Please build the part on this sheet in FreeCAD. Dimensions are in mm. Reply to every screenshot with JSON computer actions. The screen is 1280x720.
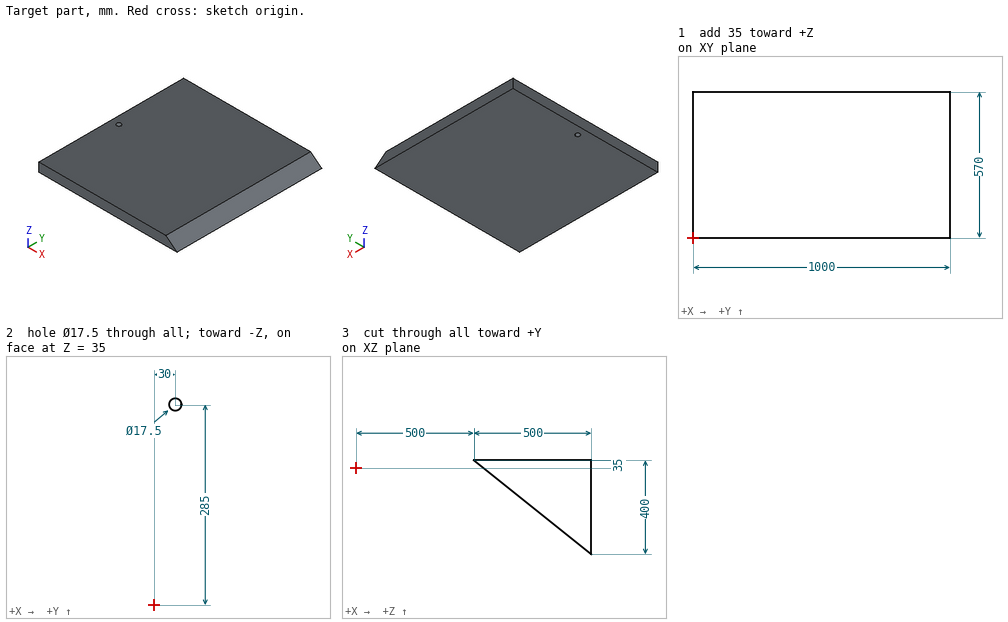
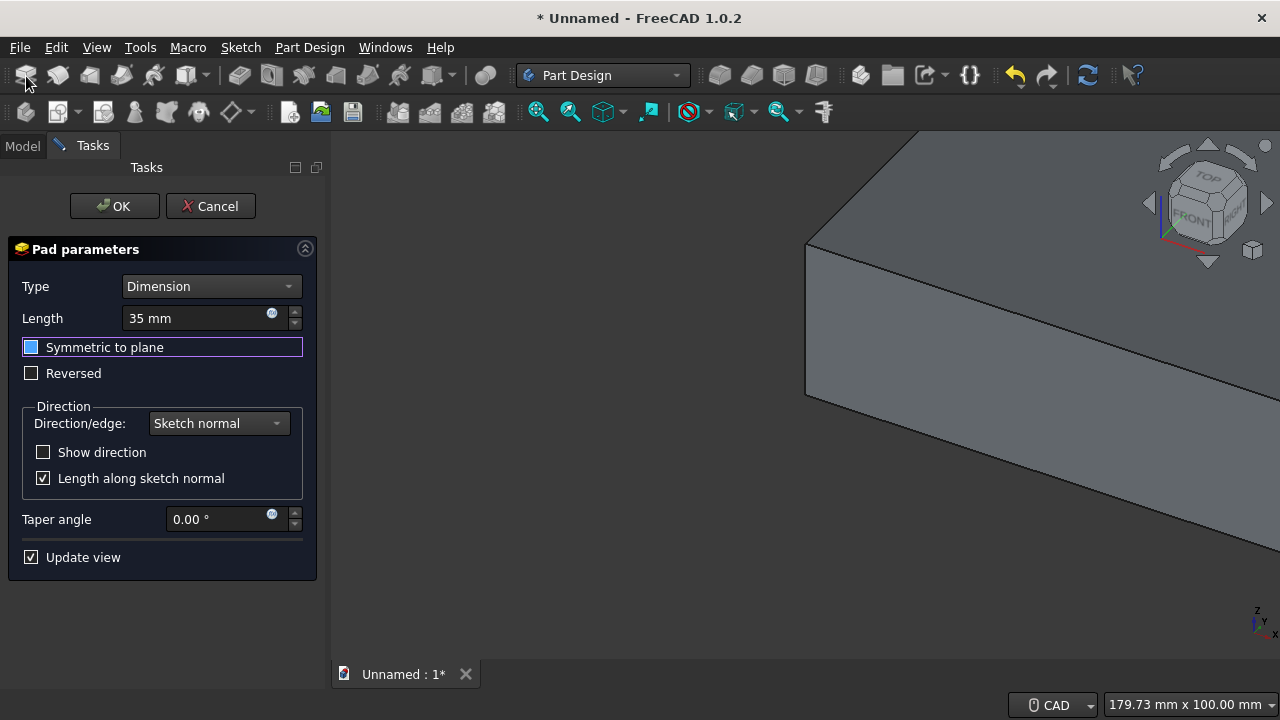
{"action": "left_click", "coordinate": [115, 206]}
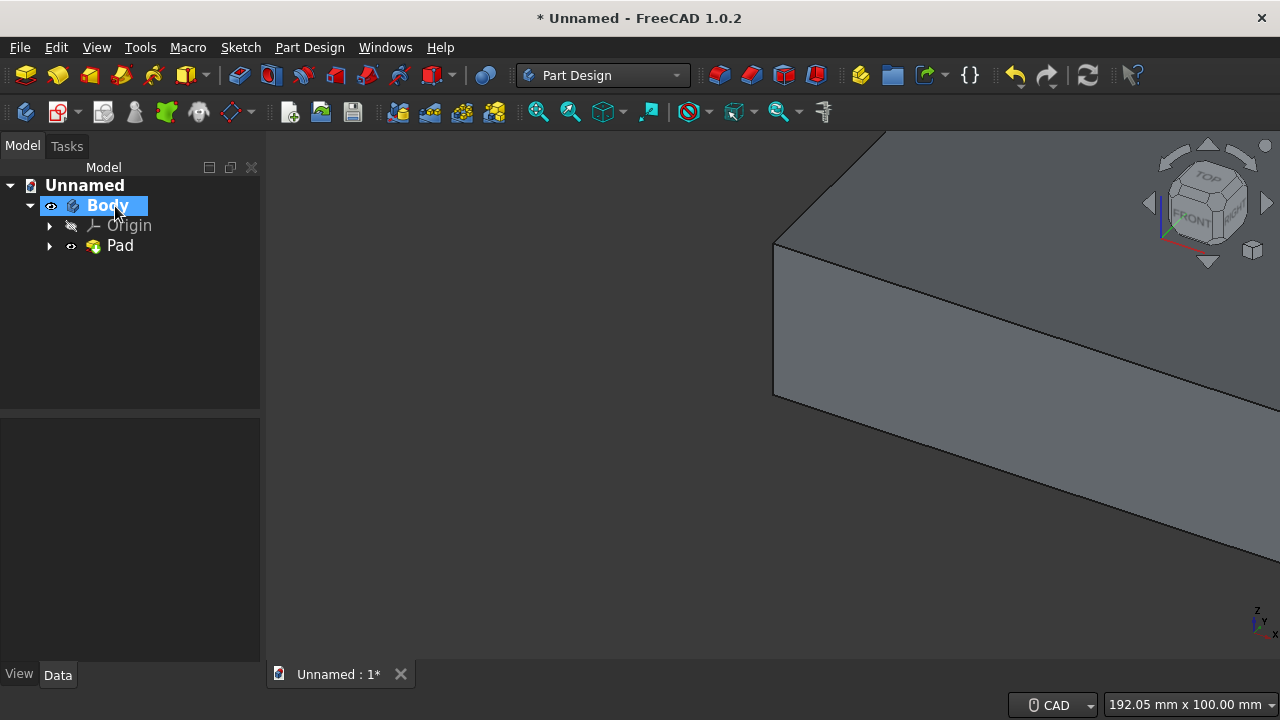
{"action": "key", "text": "v f"}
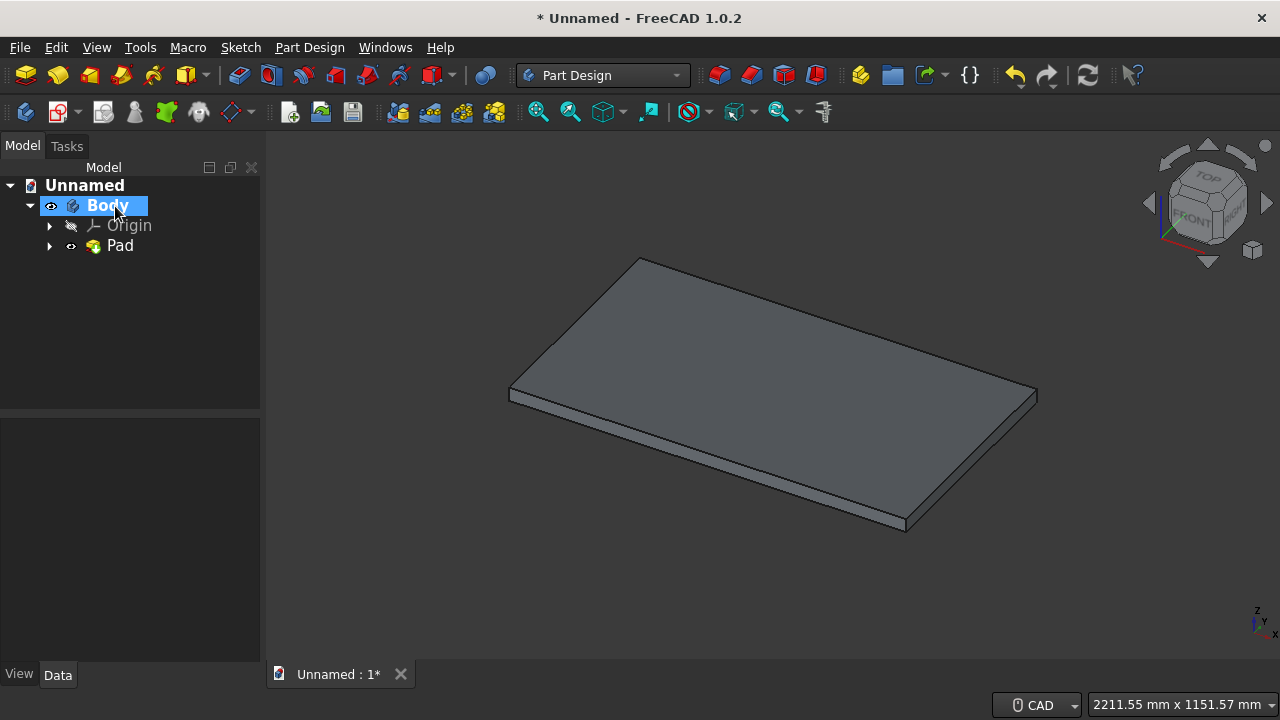
{"action": "left_click", "coordinate": [830, 406]}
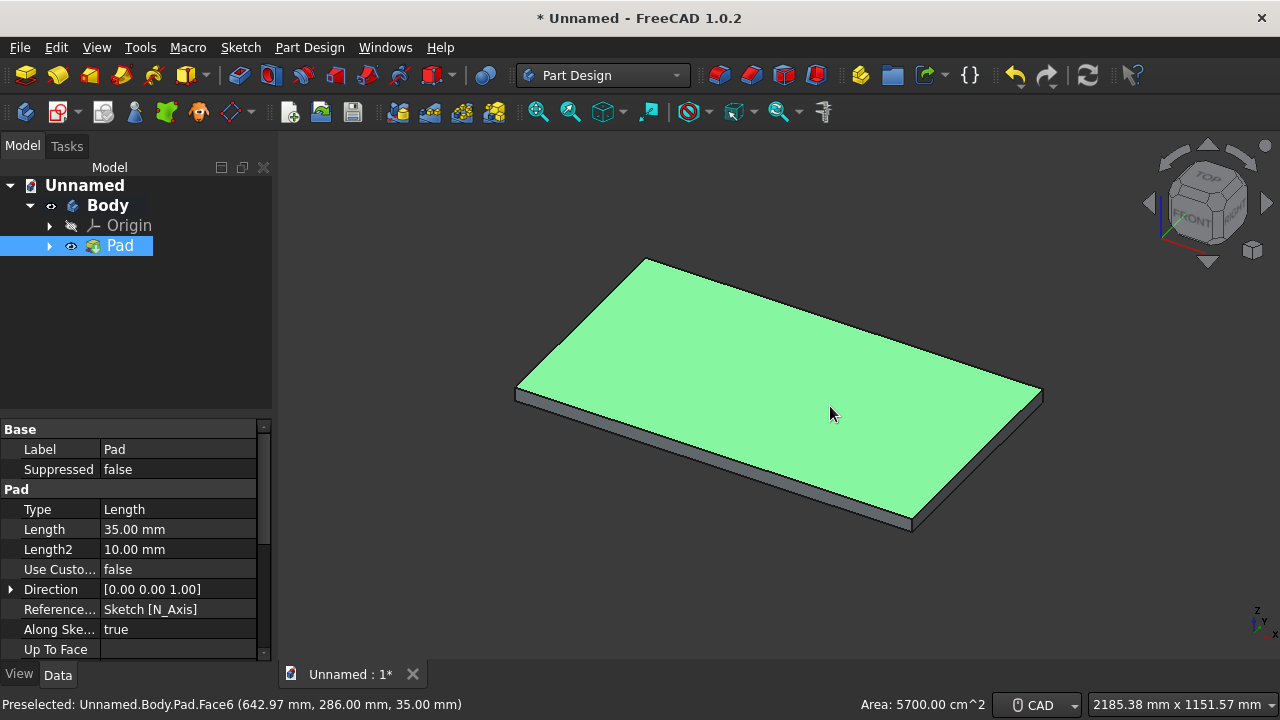
{"action": "left_click", "coordinate": [58, 112]}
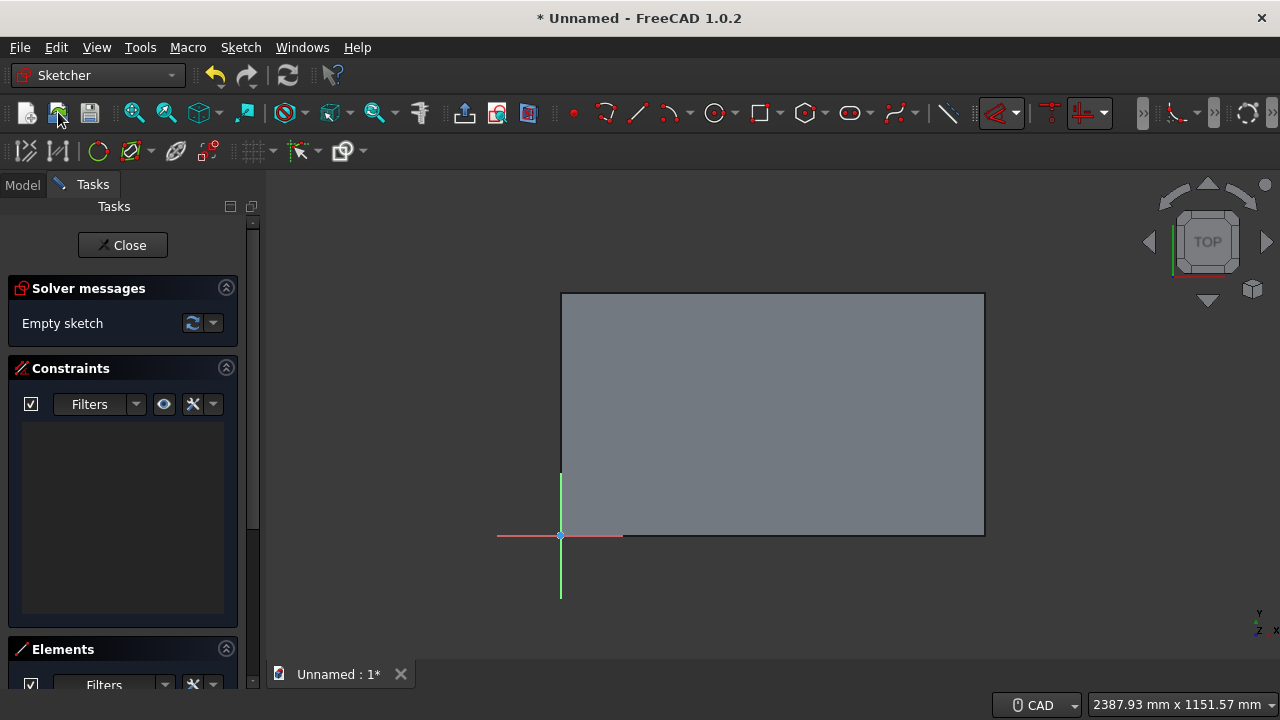
{"action": "scroll", "coordinate": [567, 414], "scroll_direction": "up", "scroll_amount": 15}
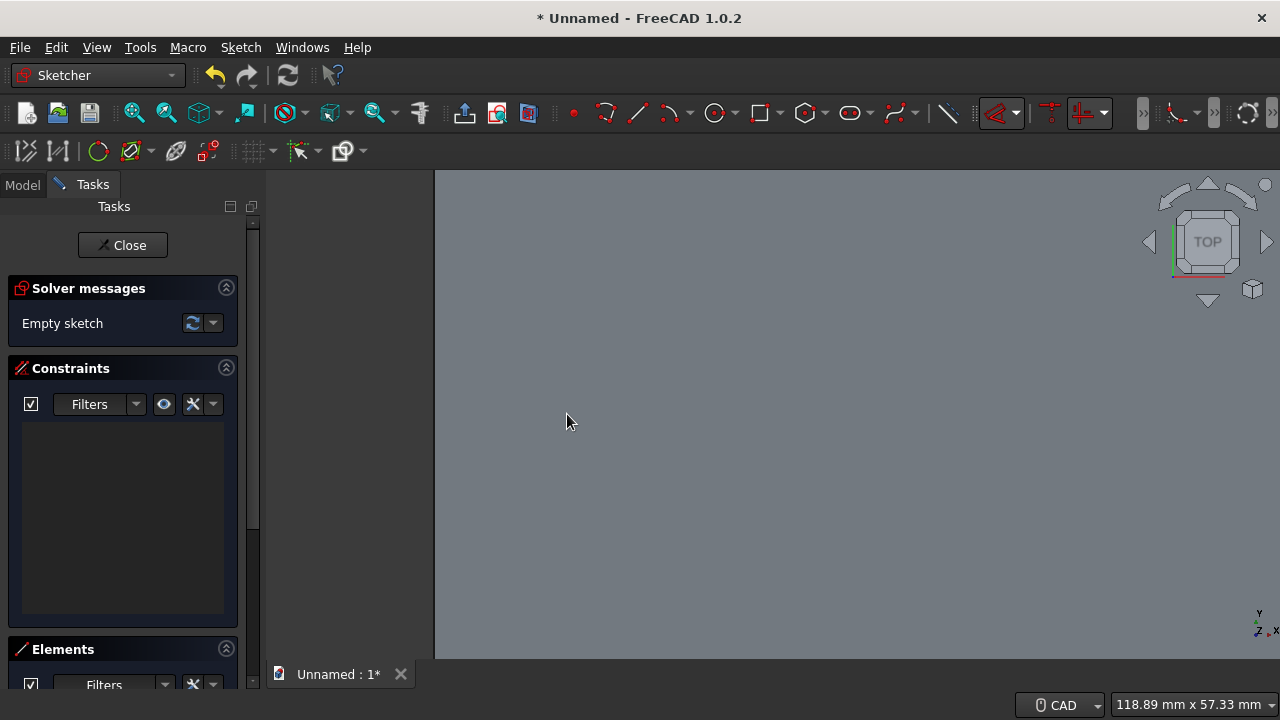
{"action": "scroll", "coordinate": [679, 414], "scroll_direction": "up", "scroll_amount": 4}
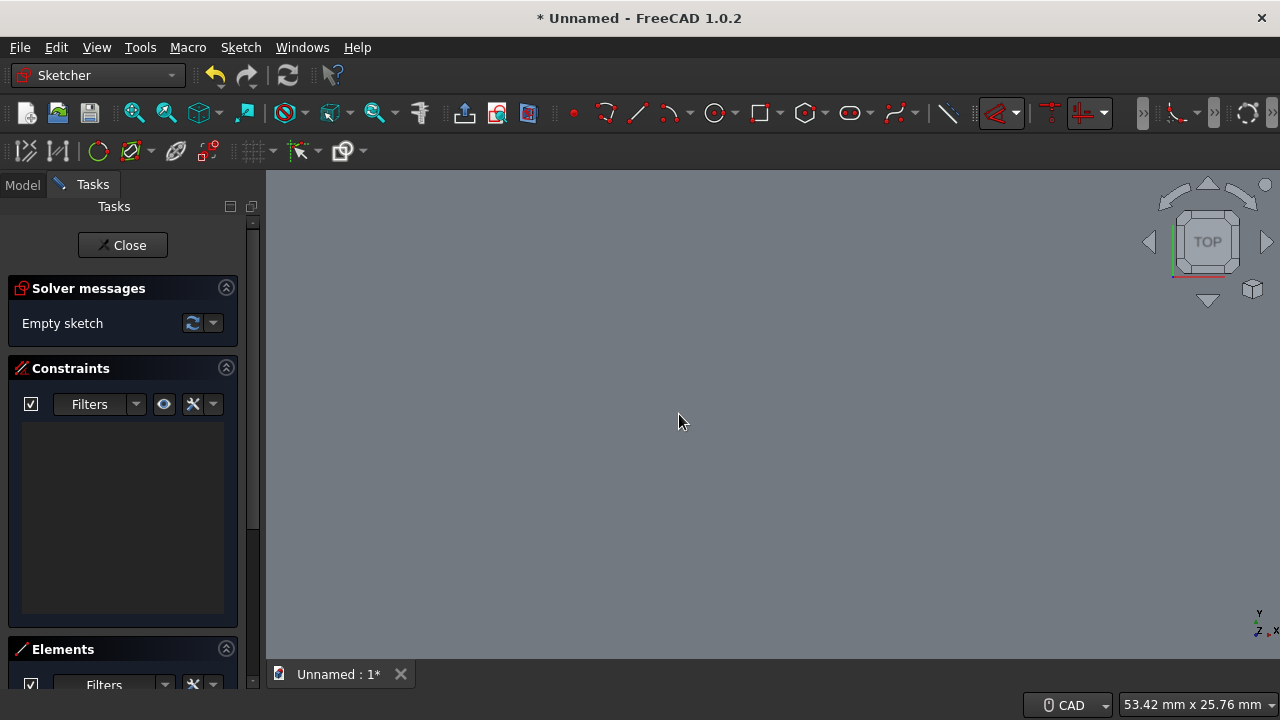
{"action": "left_click", "coordinate": [716, 114]}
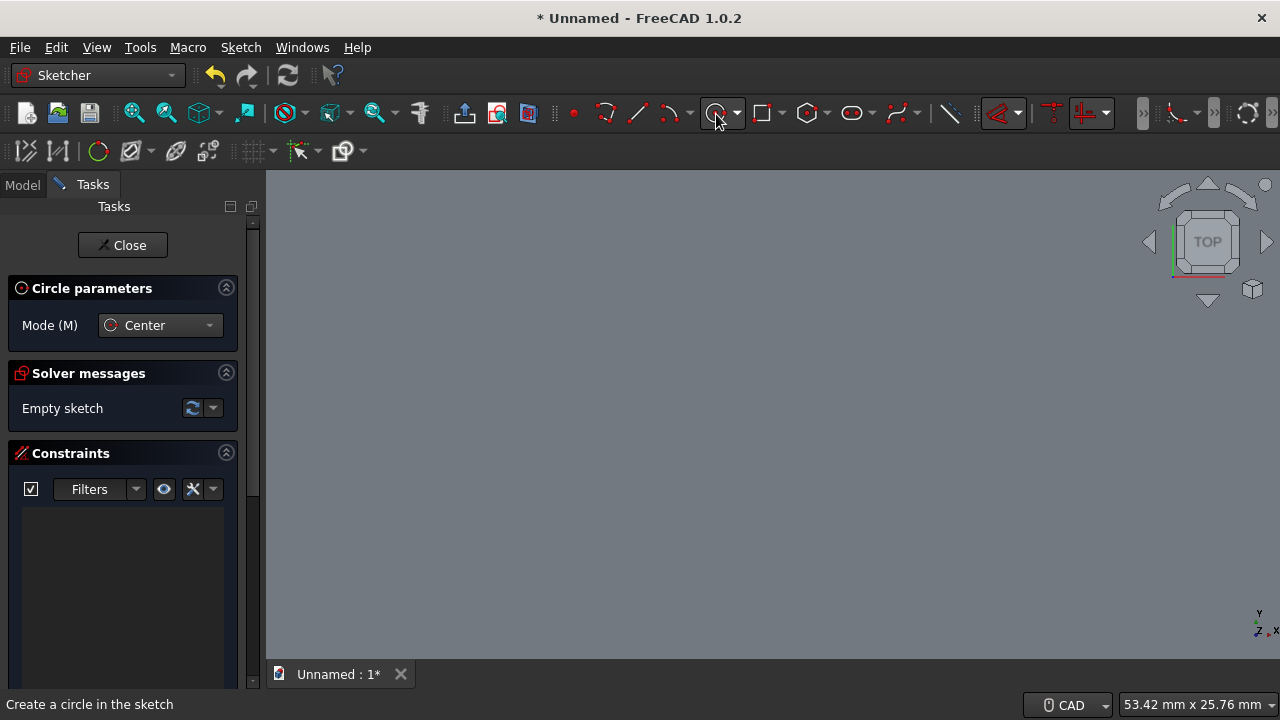
{"action": "left_click", "coordinate": [704, 414]}
{"action": "mouse_move", "coordinate": [821, 297]}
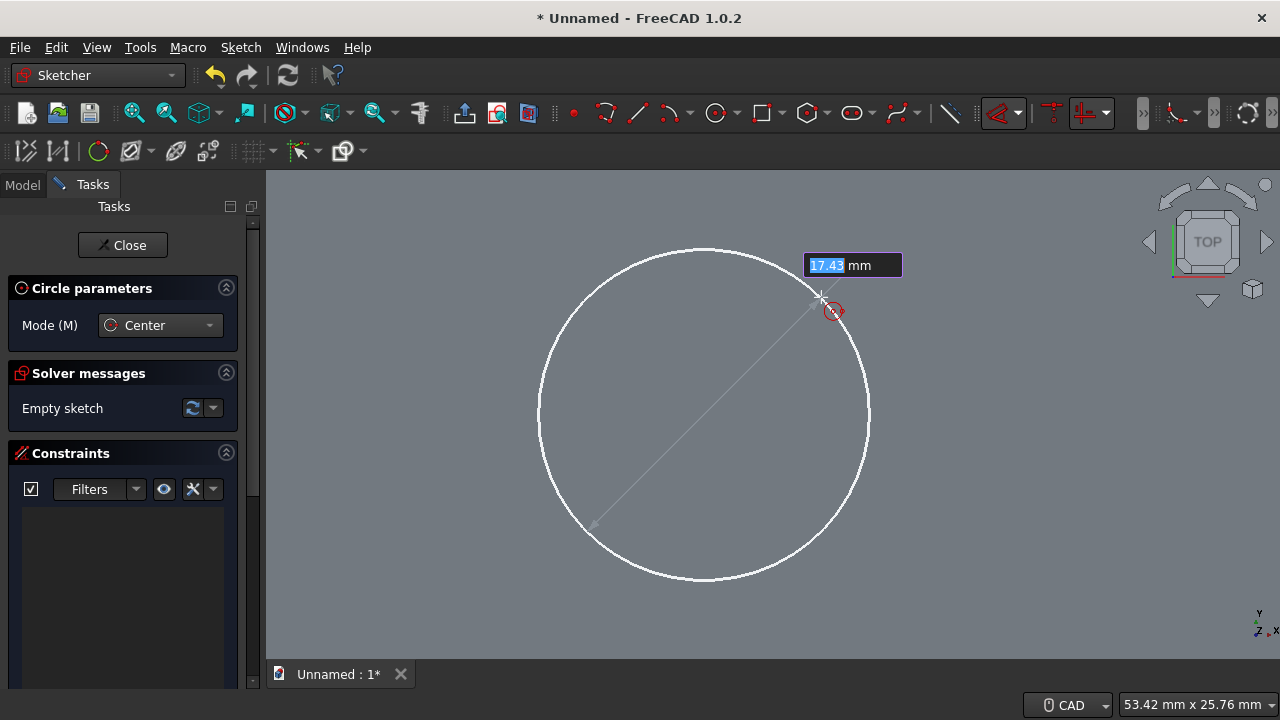
{"action": "type", "text": "17.5"}
{"action": "key", "text": "Return"}
{"action": "key", "text": "Escape"}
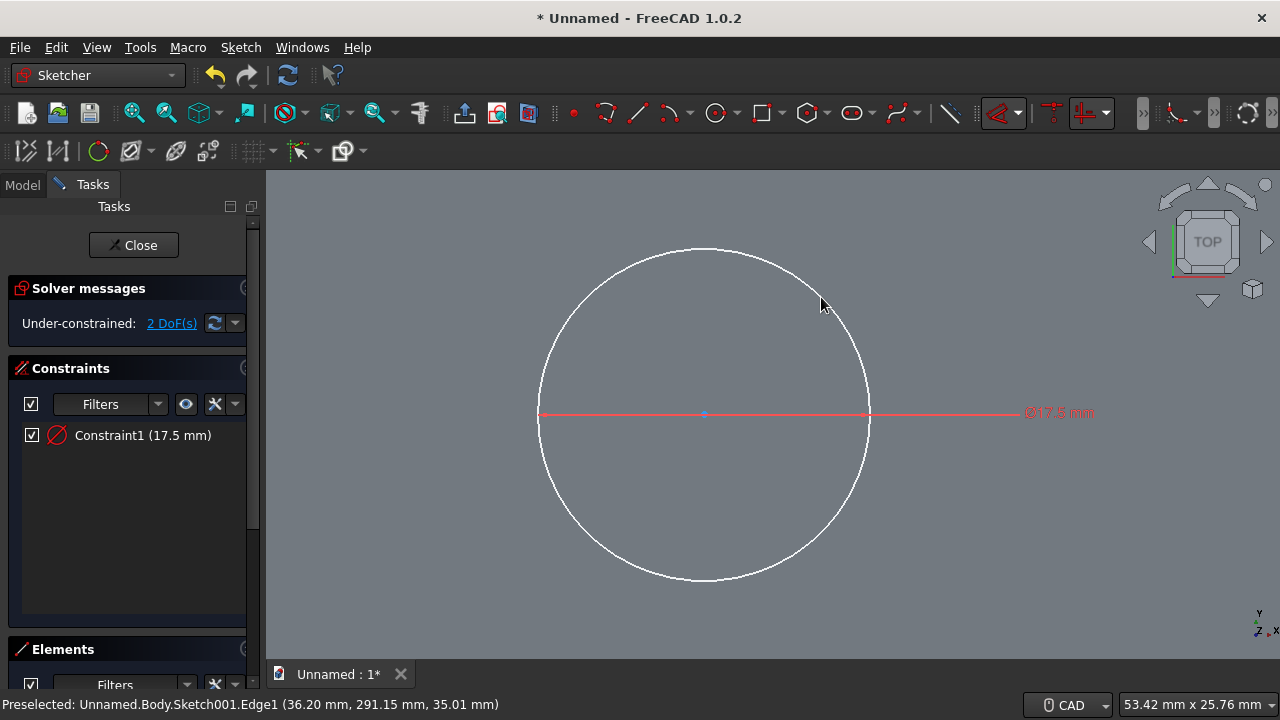
{"action": "left_click", "coordinate": [998, 114]}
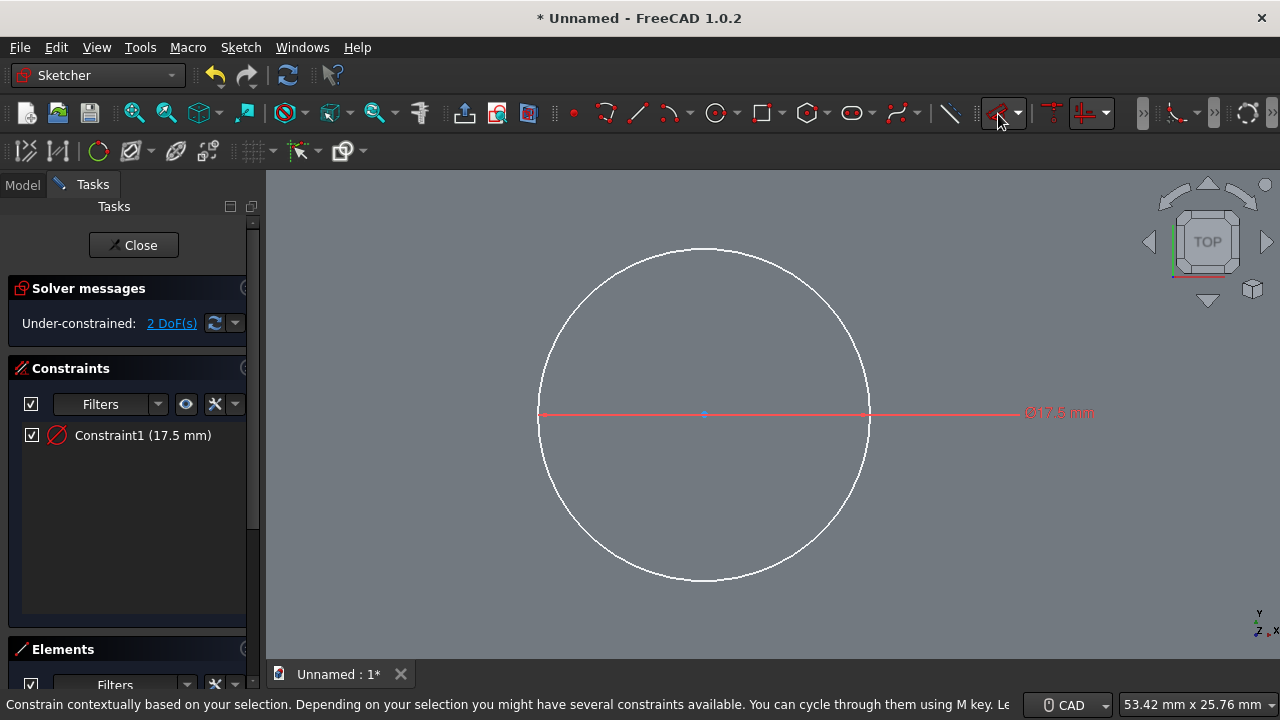
{"action": "left_click", "coordinate": [704, 415]}
{"action": "left_click", "coordinate": [499, 381]}